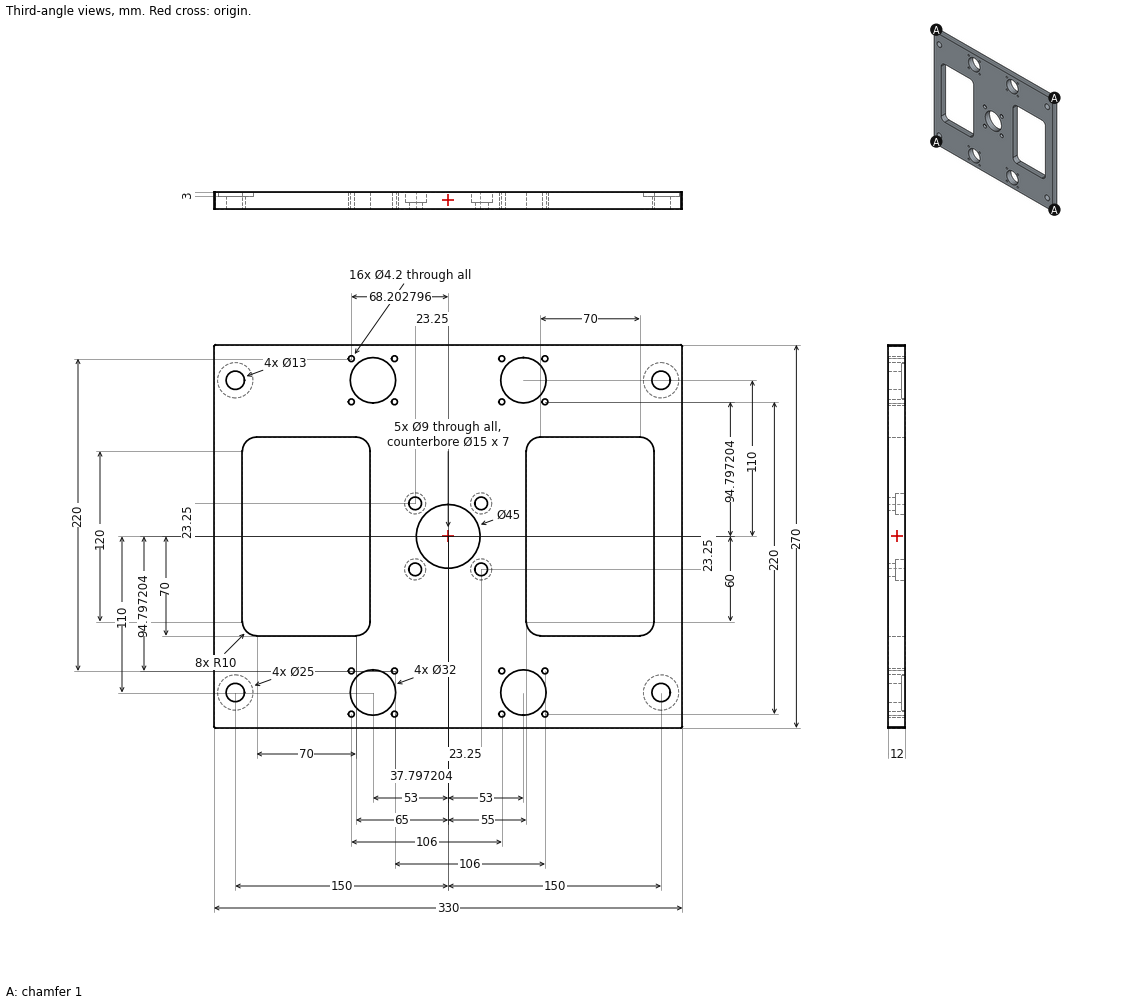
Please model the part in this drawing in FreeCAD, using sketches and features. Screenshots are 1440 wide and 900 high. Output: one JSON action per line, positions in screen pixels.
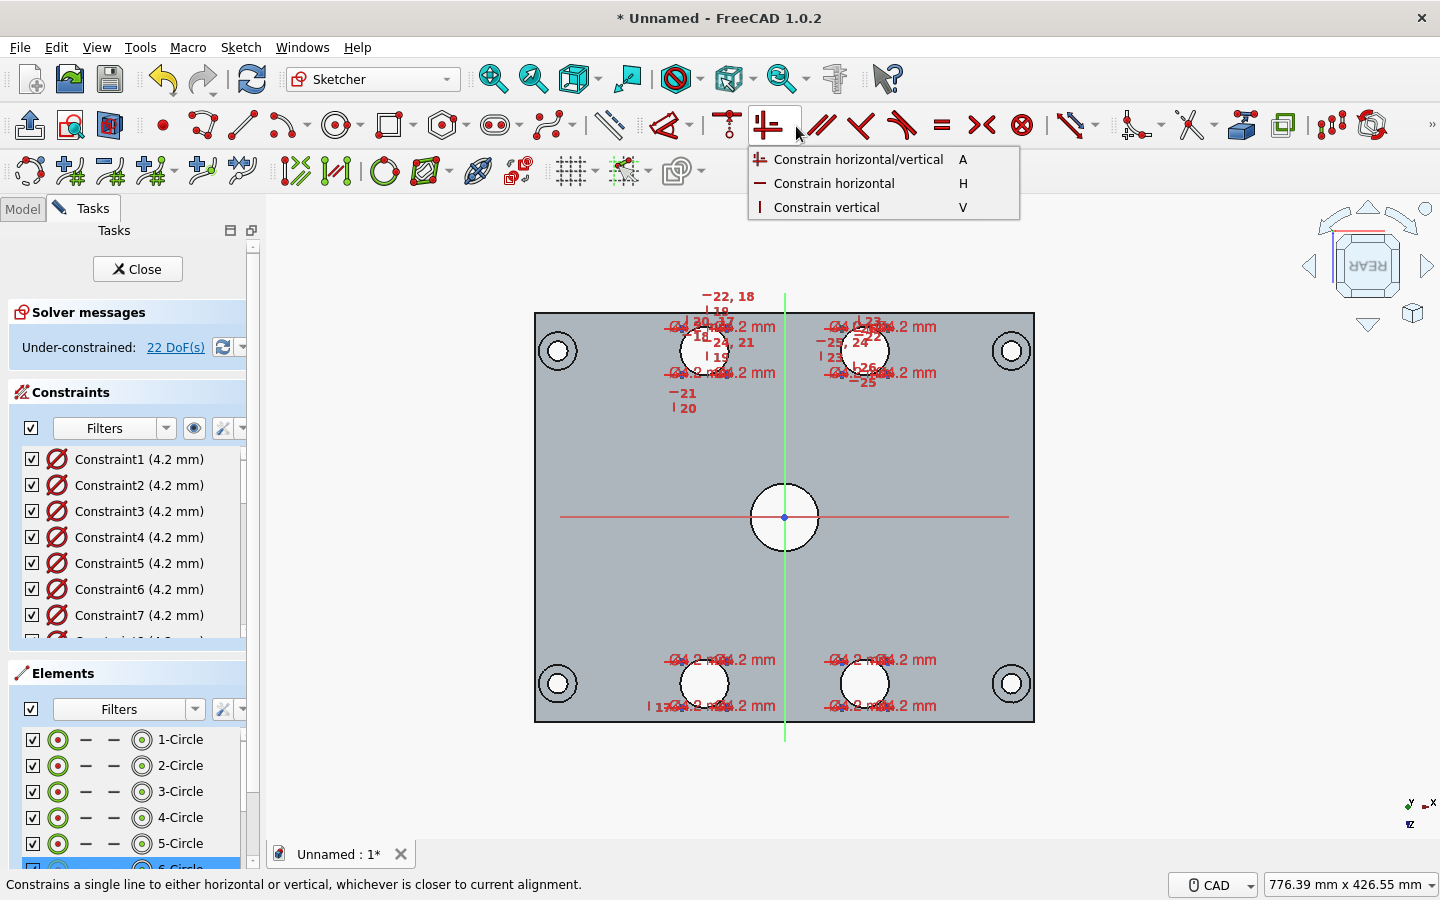
{"action": "left_click", "coordinate": [884, 183]}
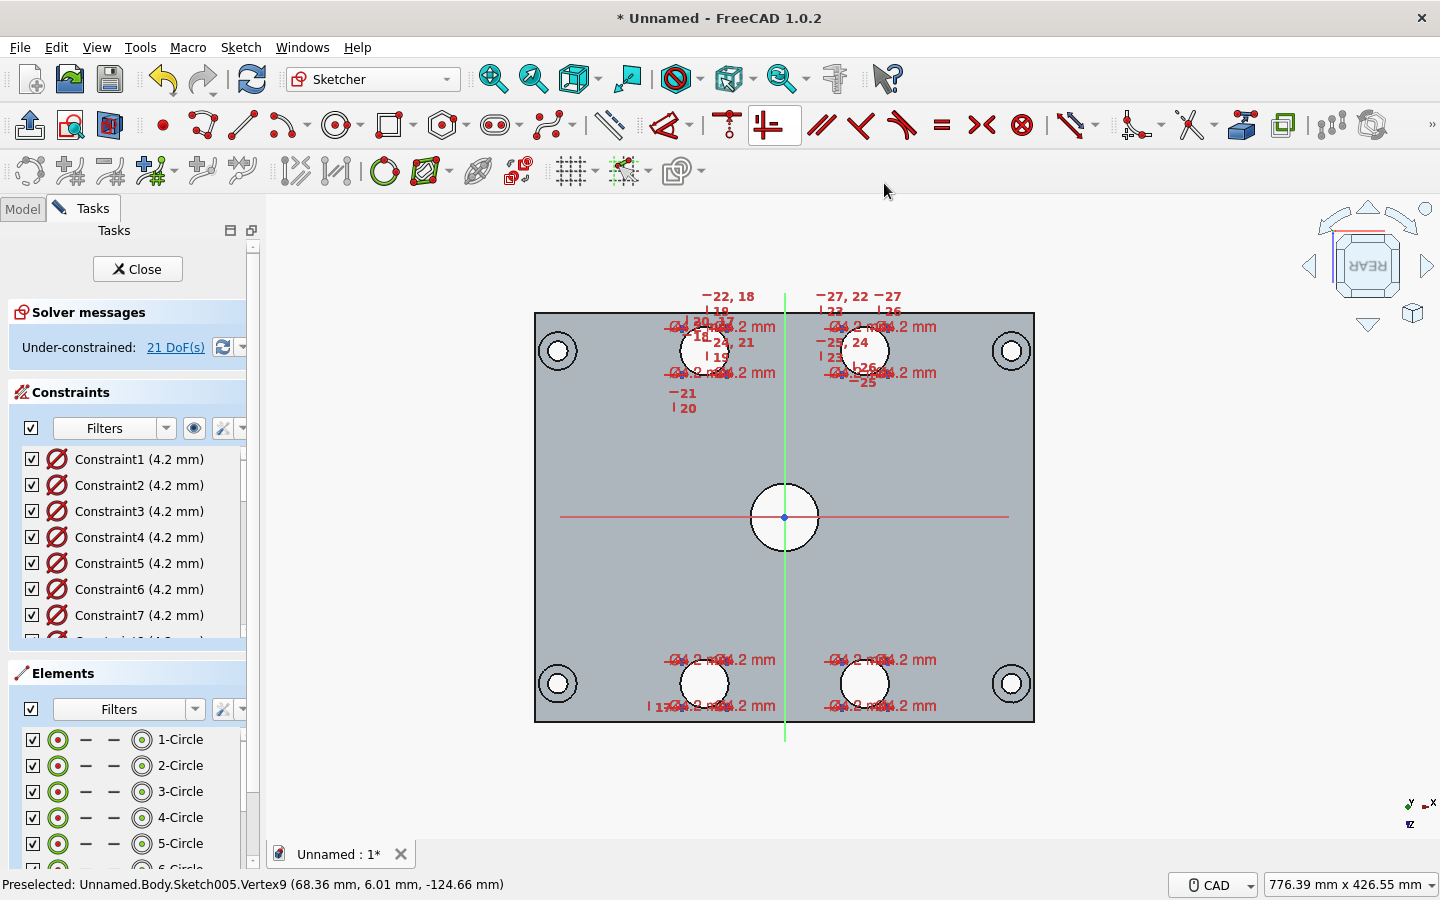
{"action": "left_click", "coordinate": [888, 375]}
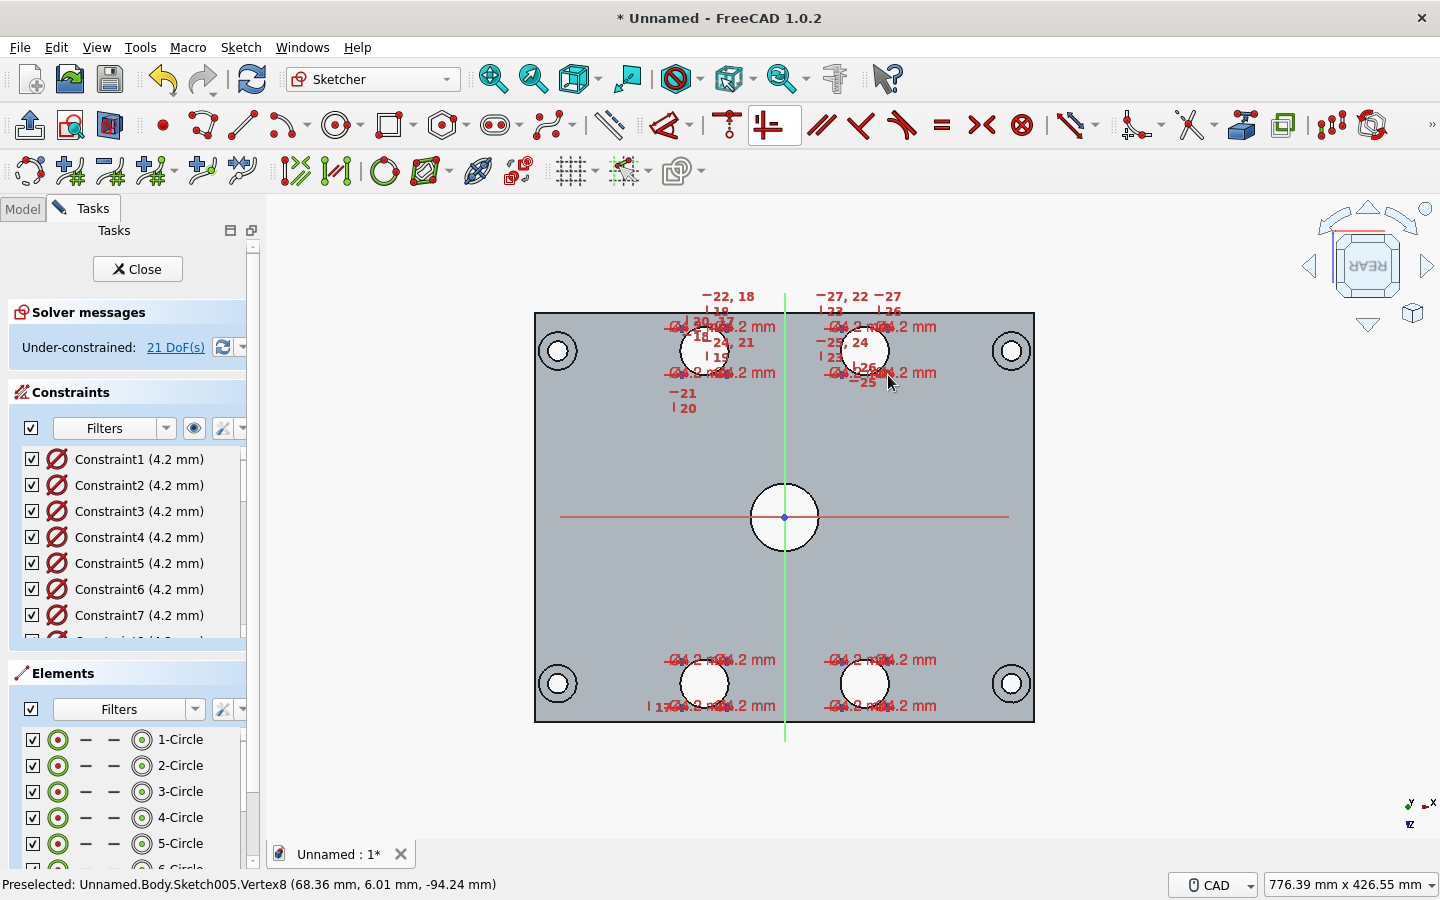
{"action": "left_click", "coordinate": [888, 708]}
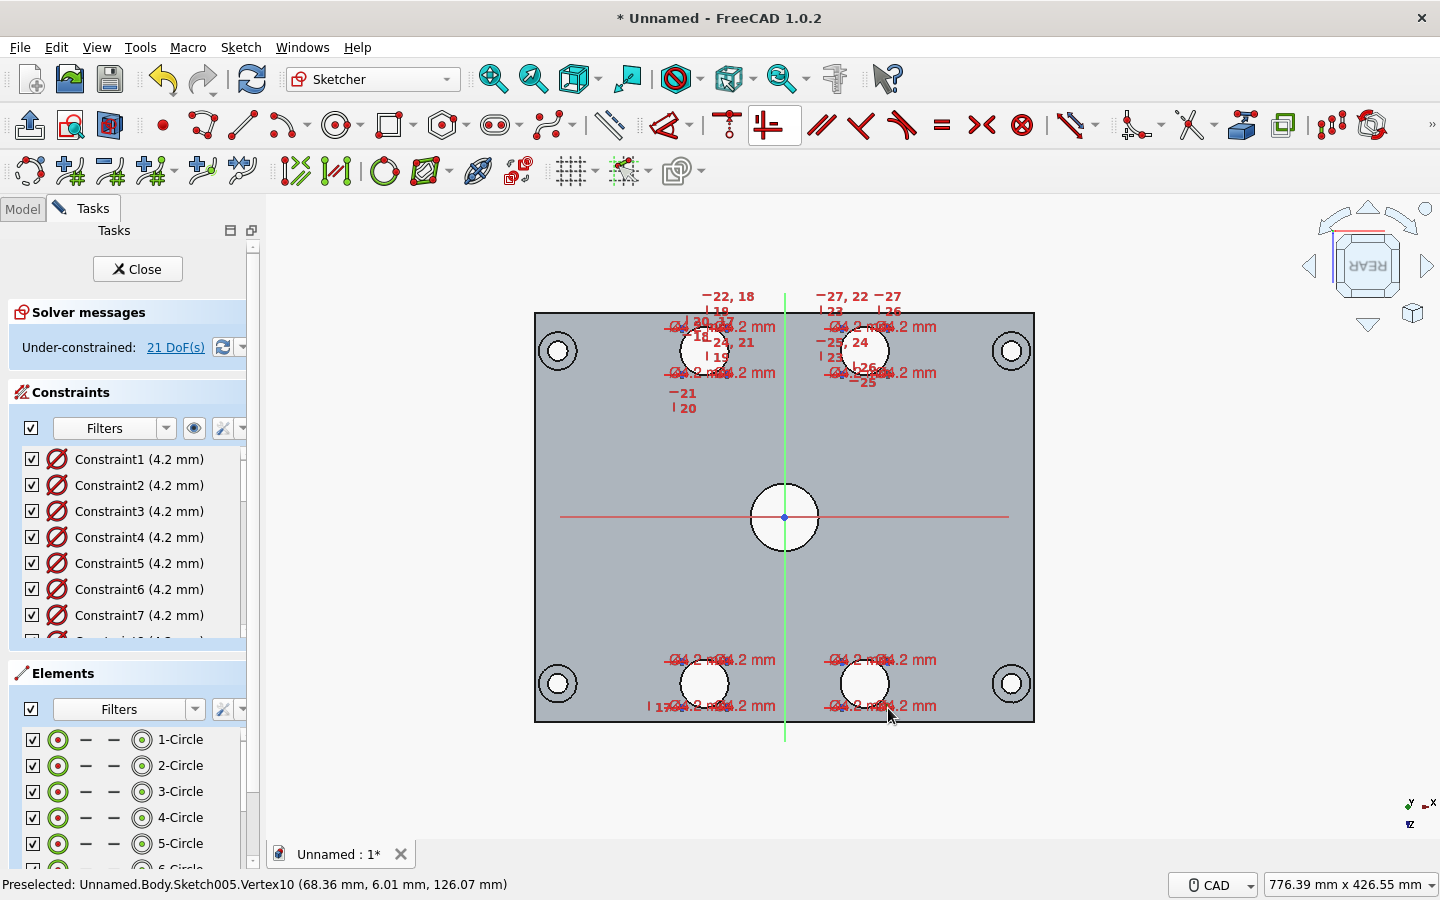
{"action": "left_click", "coordinate": [796, 126]}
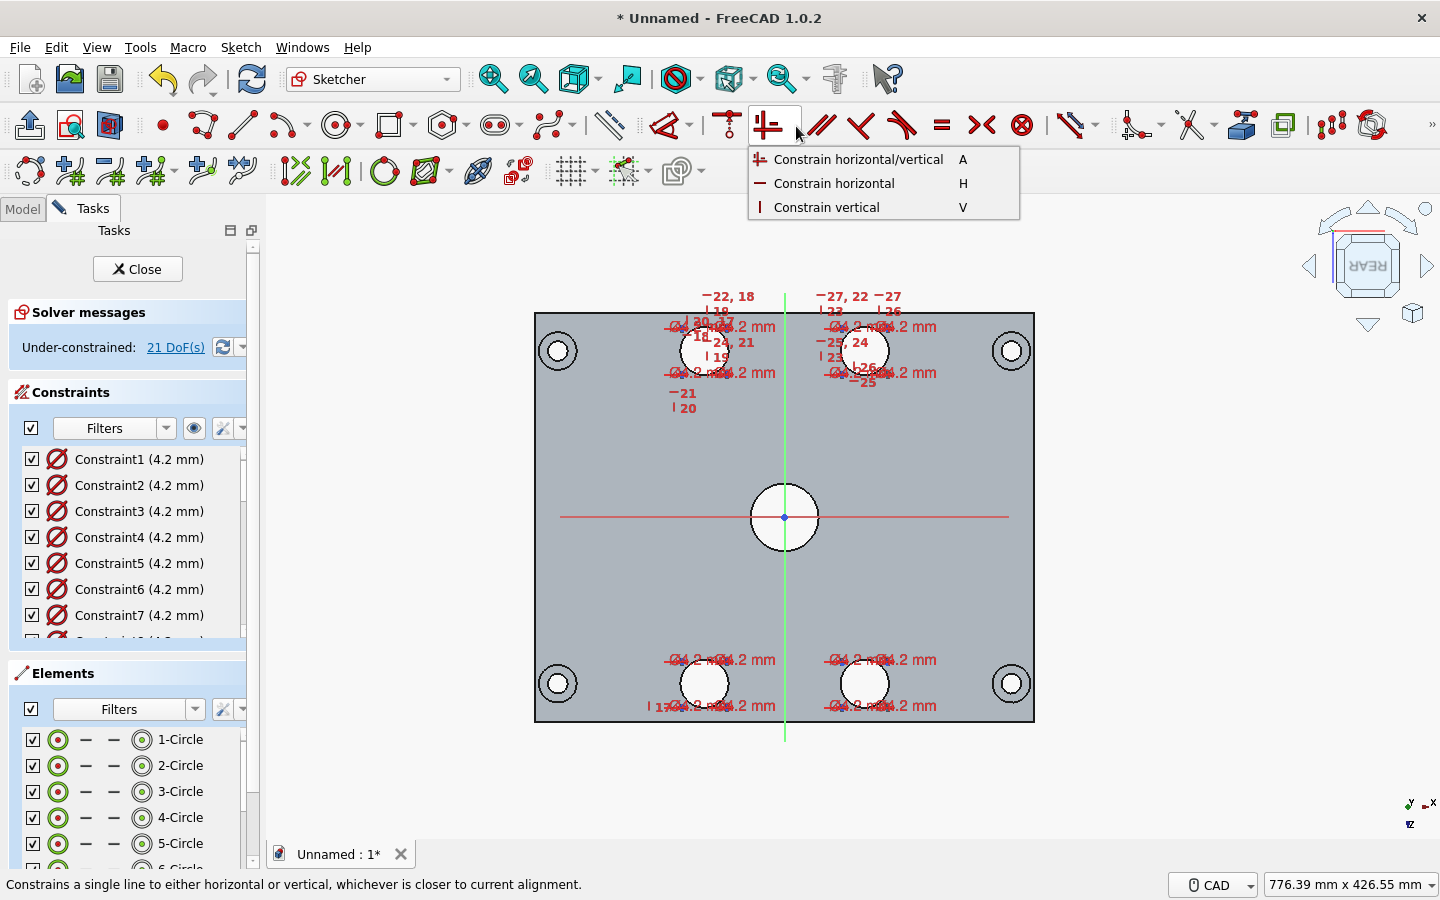
{"action": "left_click", "coordinate": [884, 207]}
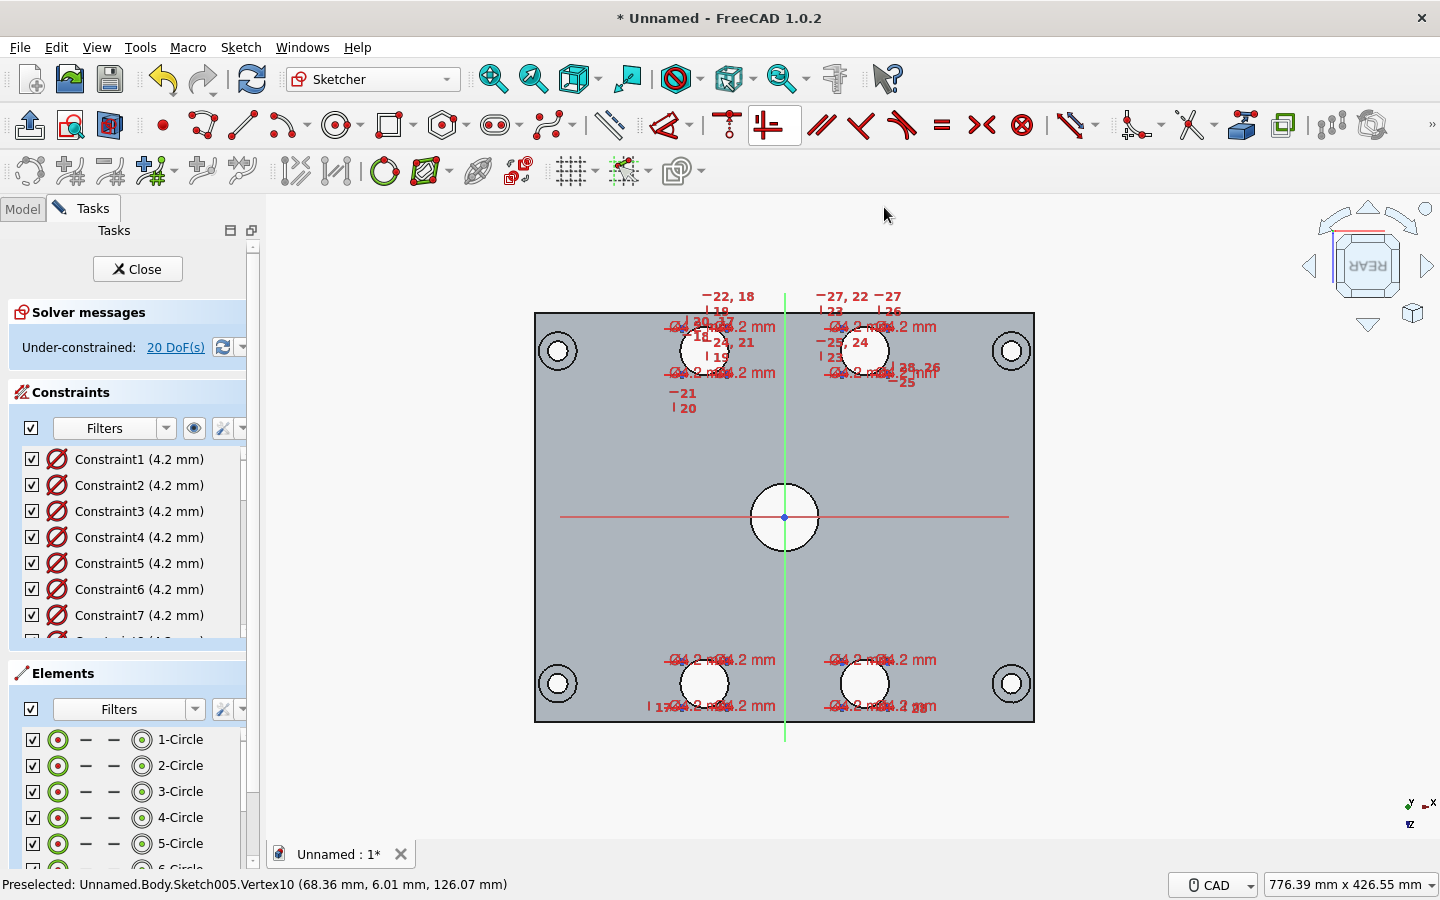
{"action": "left_click", "coordinate": [682, 708]}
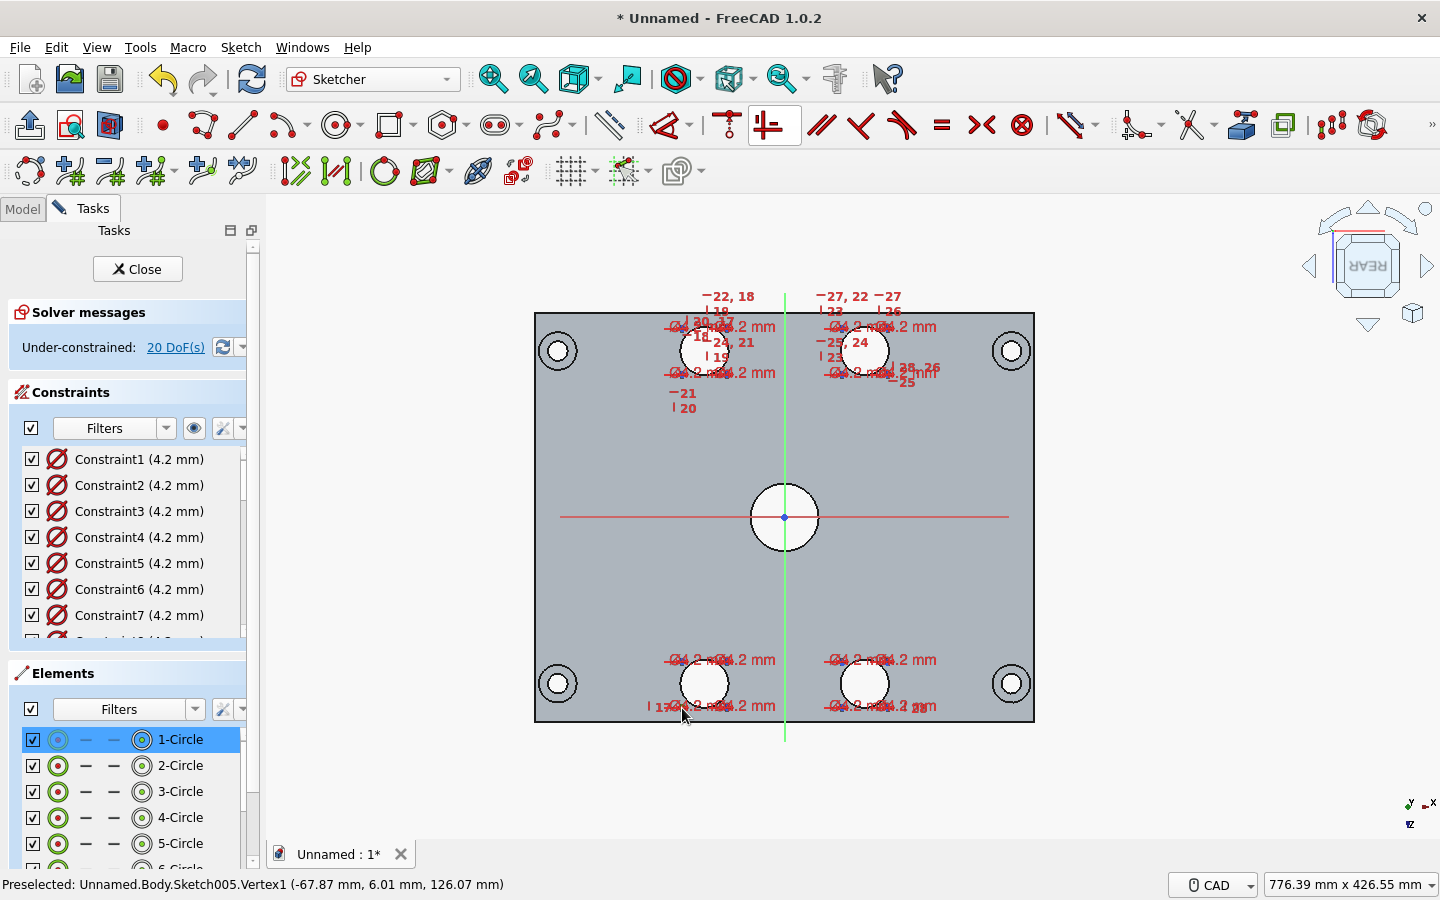
{"action": "left_click", "coordinate": [888, 708]}